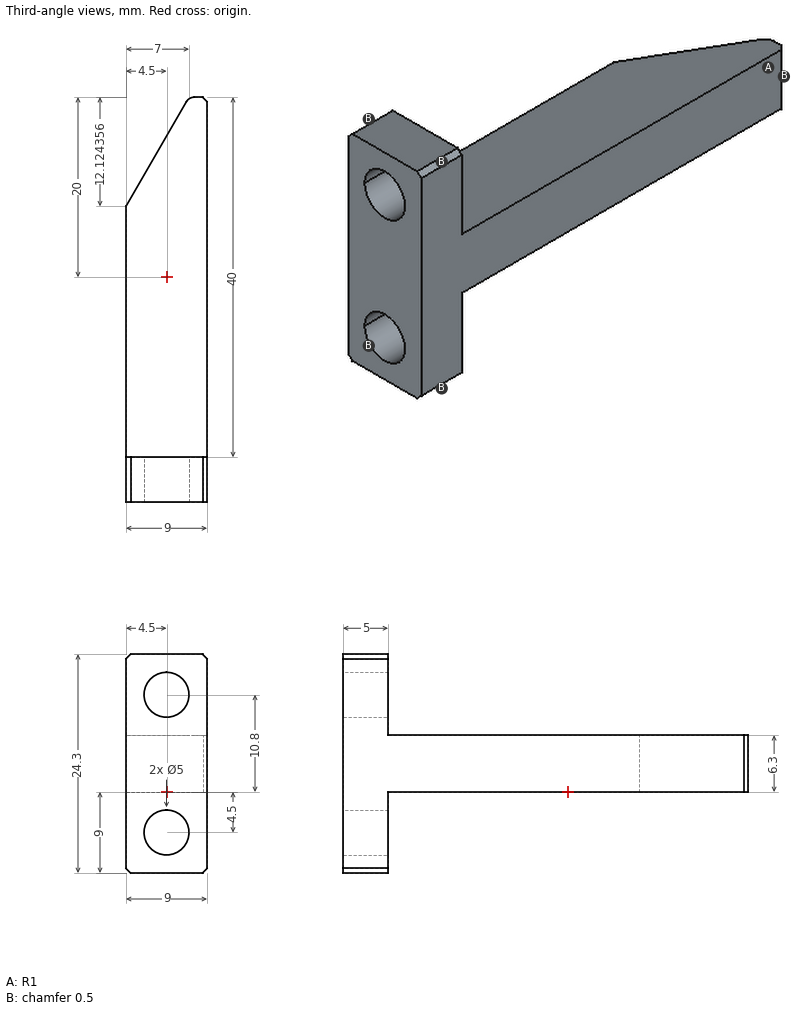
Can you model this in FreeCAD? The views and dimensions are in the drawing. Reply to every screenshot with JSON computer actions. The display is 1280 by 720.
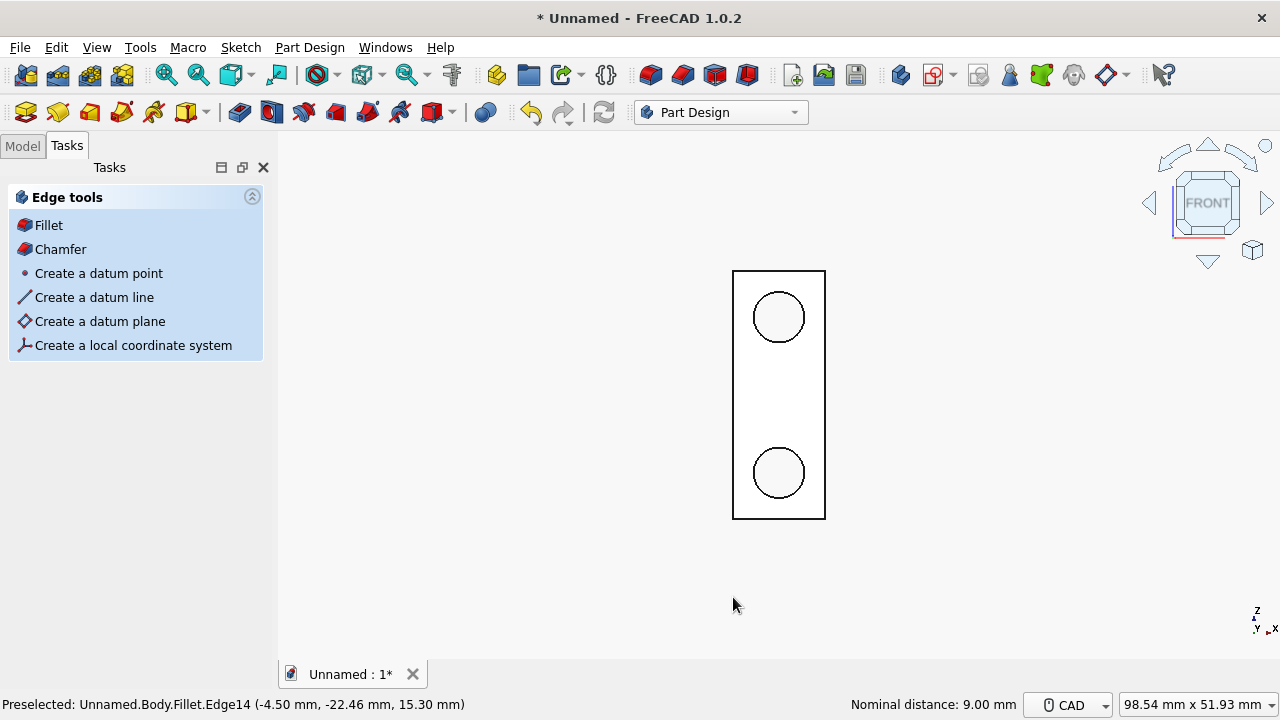
{"action": "key", "text": "3"}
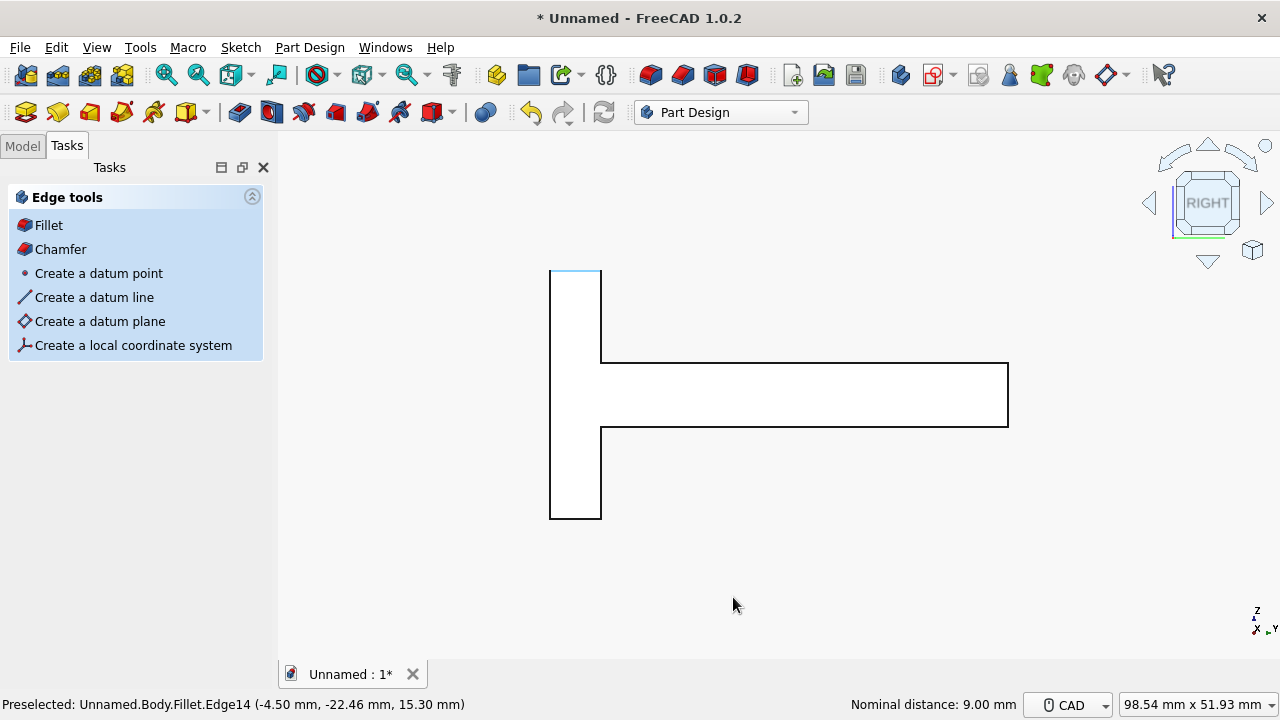
{"action": "left_click", "coordinate": [576, 518], "text": "ctrl"}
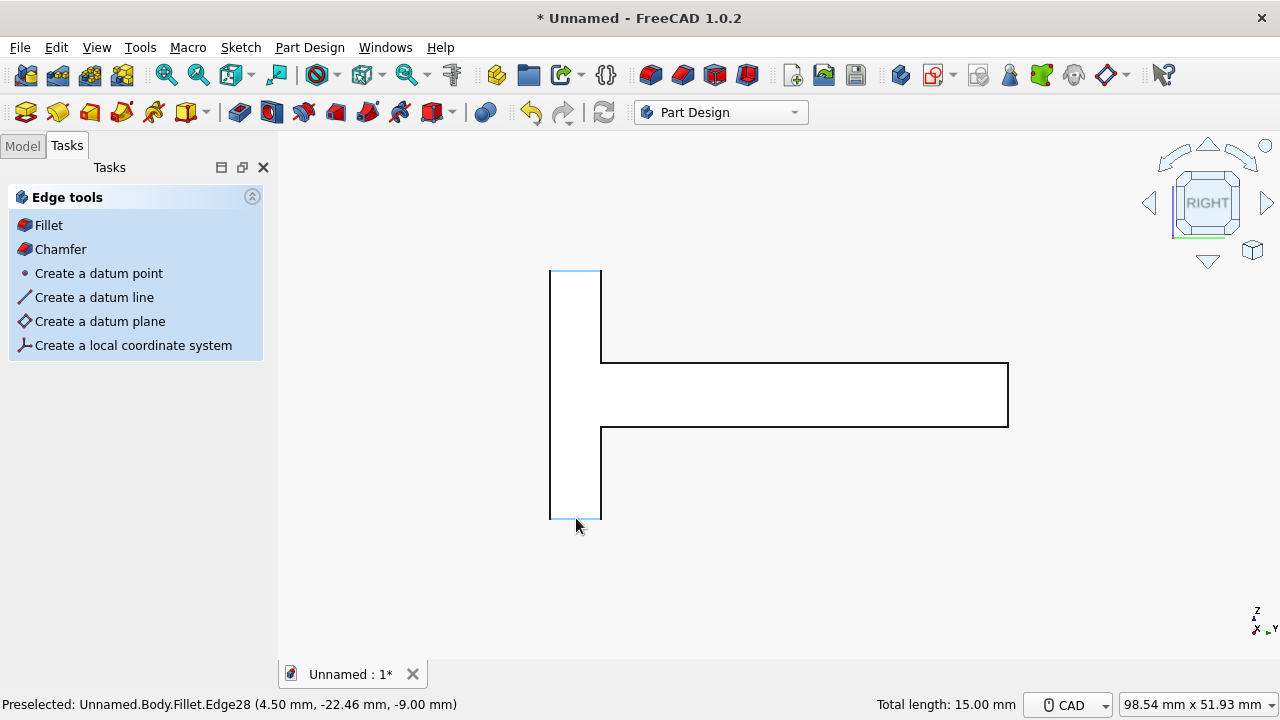
{"action": "left_click", "coordinate": [1008, 394], "text": "ctrl"}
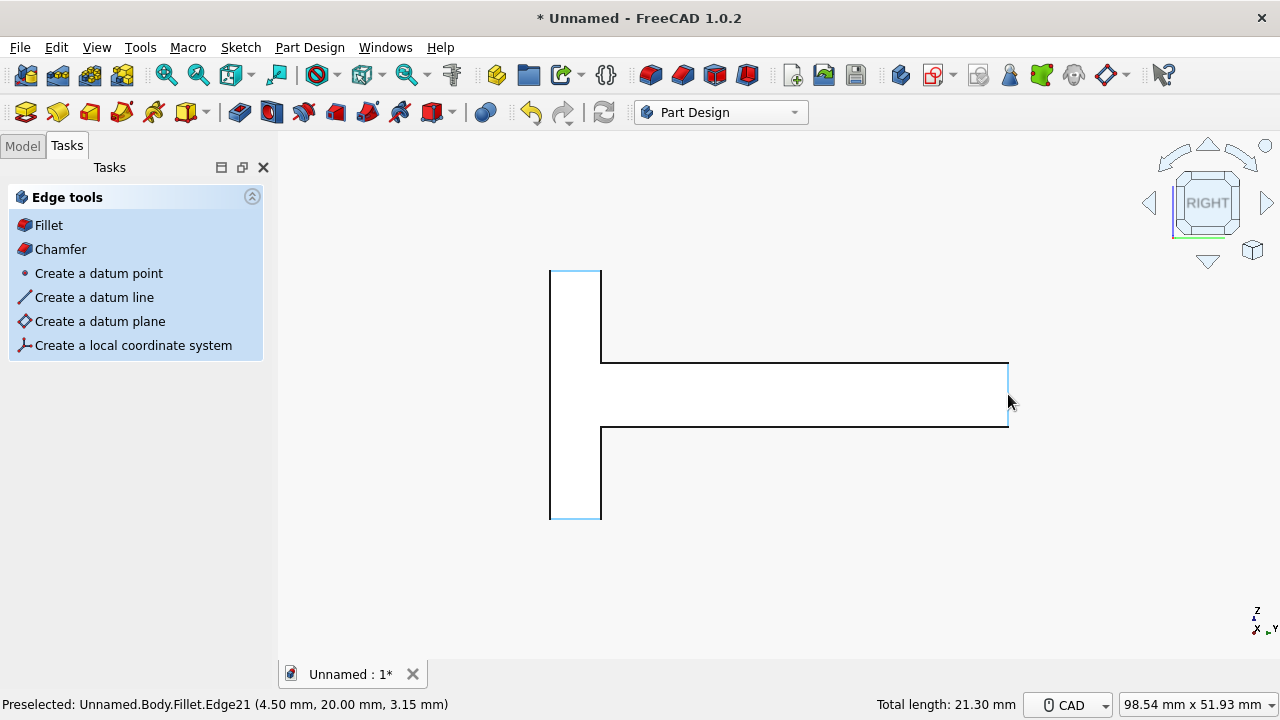
{"action": "key", "text": "5"}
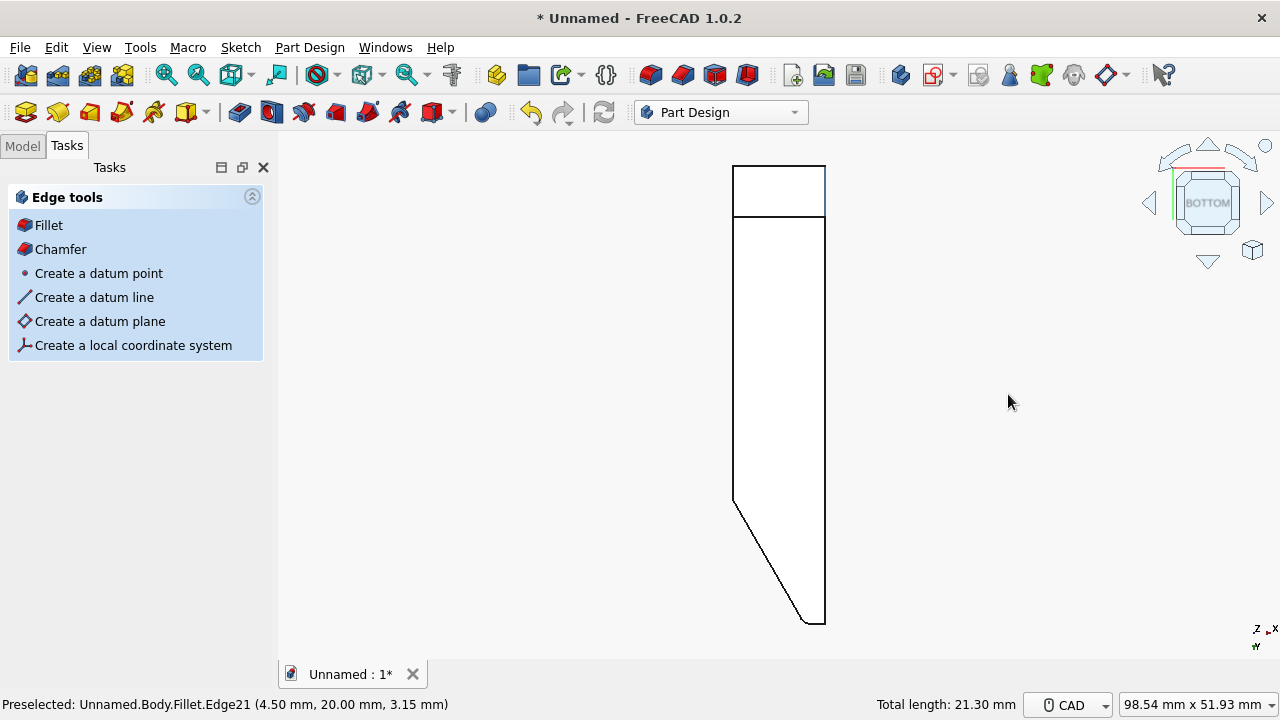
{"action": "left_click", "coordinate": [733, 191], "text": "ctrl"}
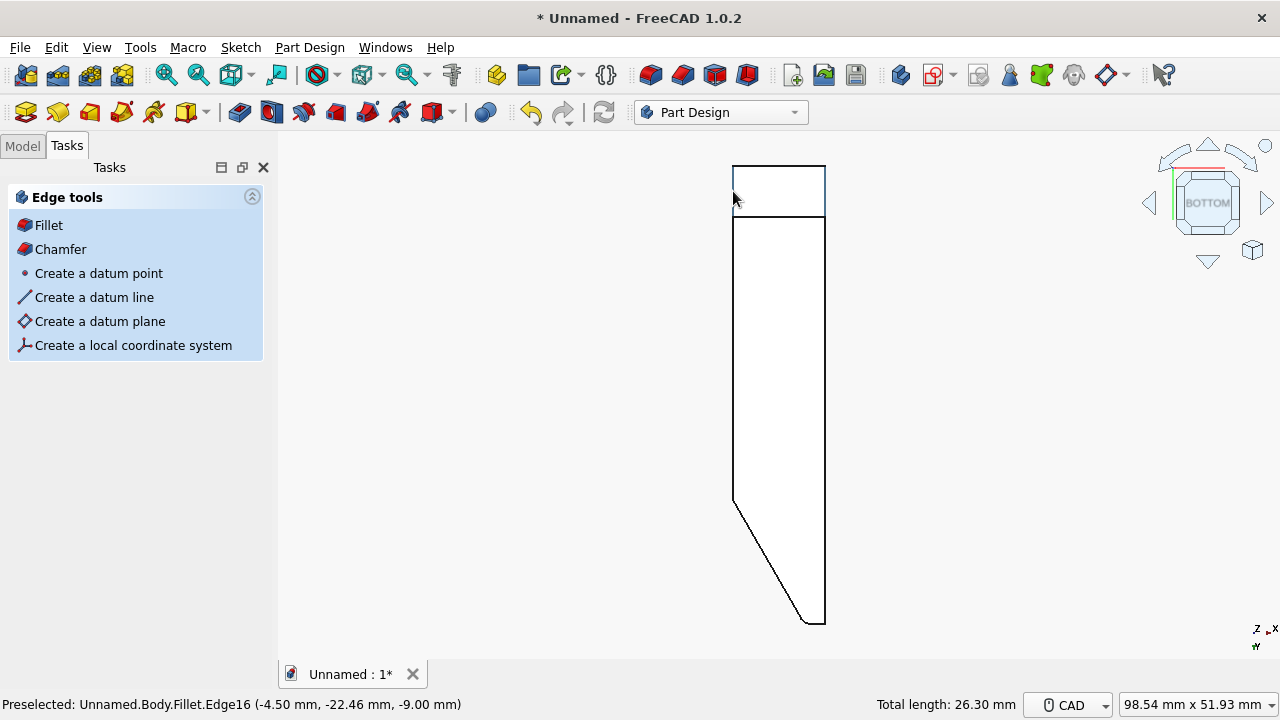
{"action": "left_click", "coordinate": [684, 76]}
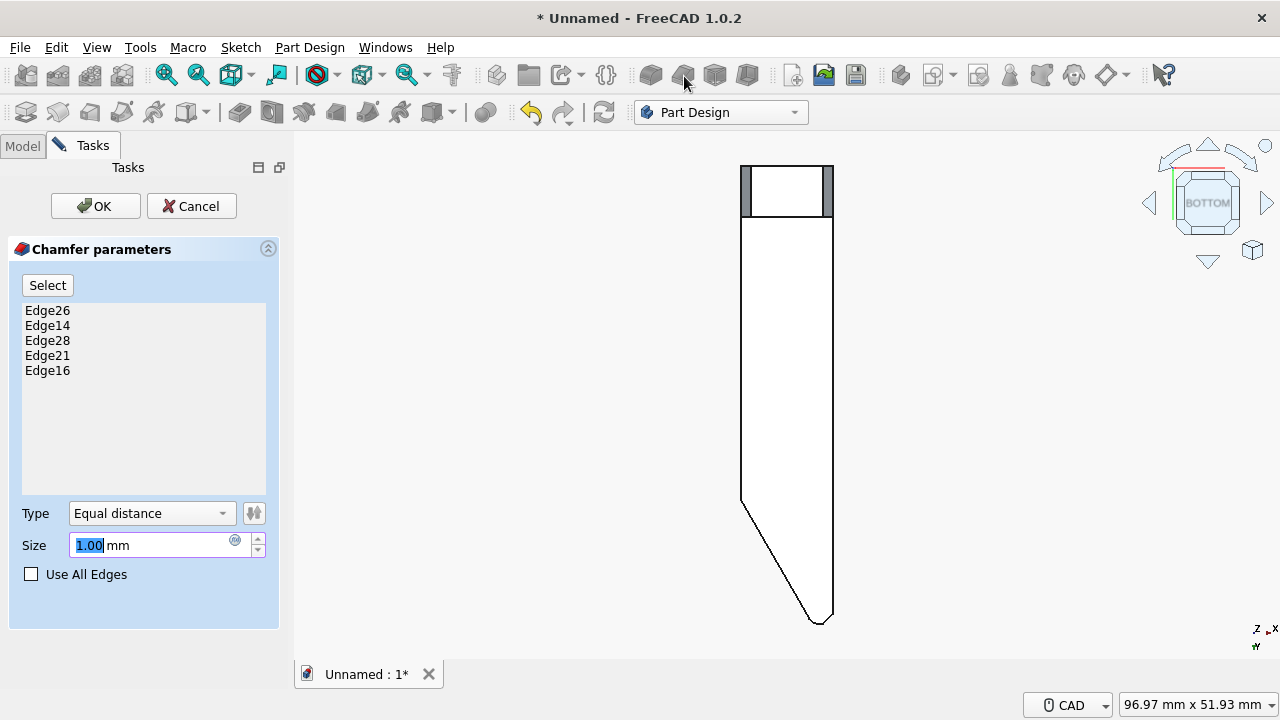
{"action": "type", "text": "0.5"}
{"action": "key", "text": "Tab"}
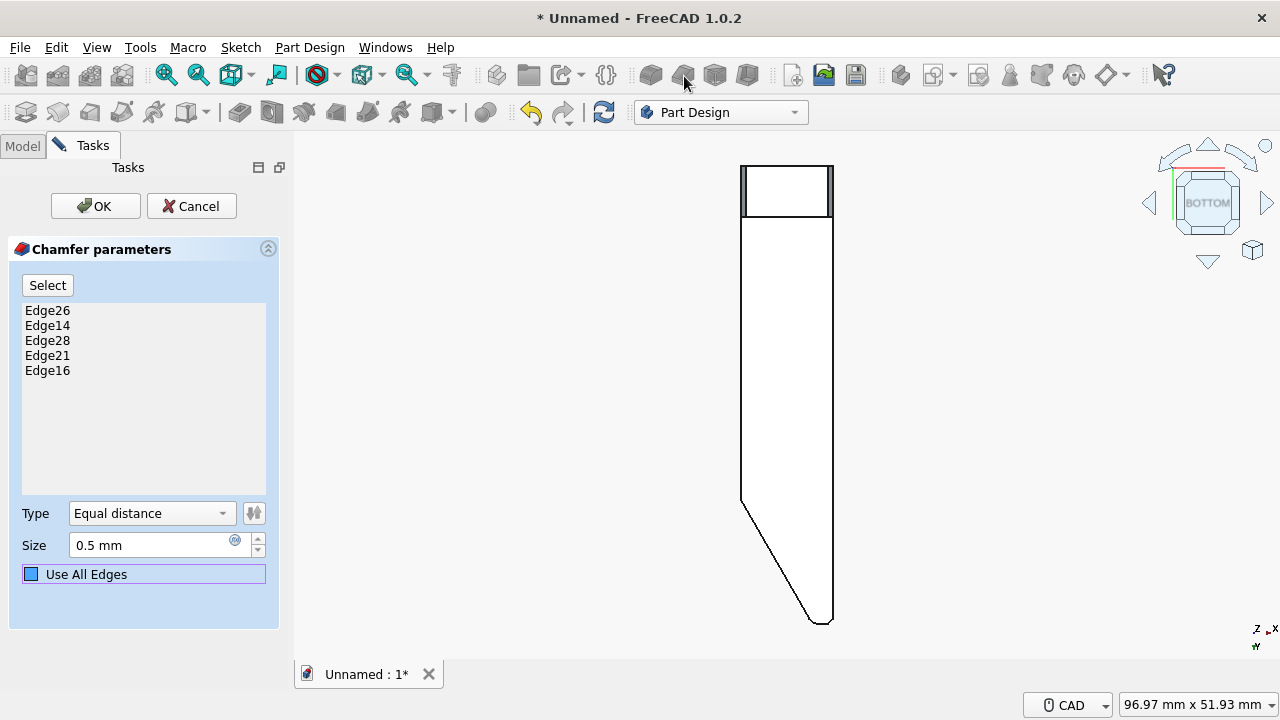
{"action": "left_click", "coordinate": [96, 206]}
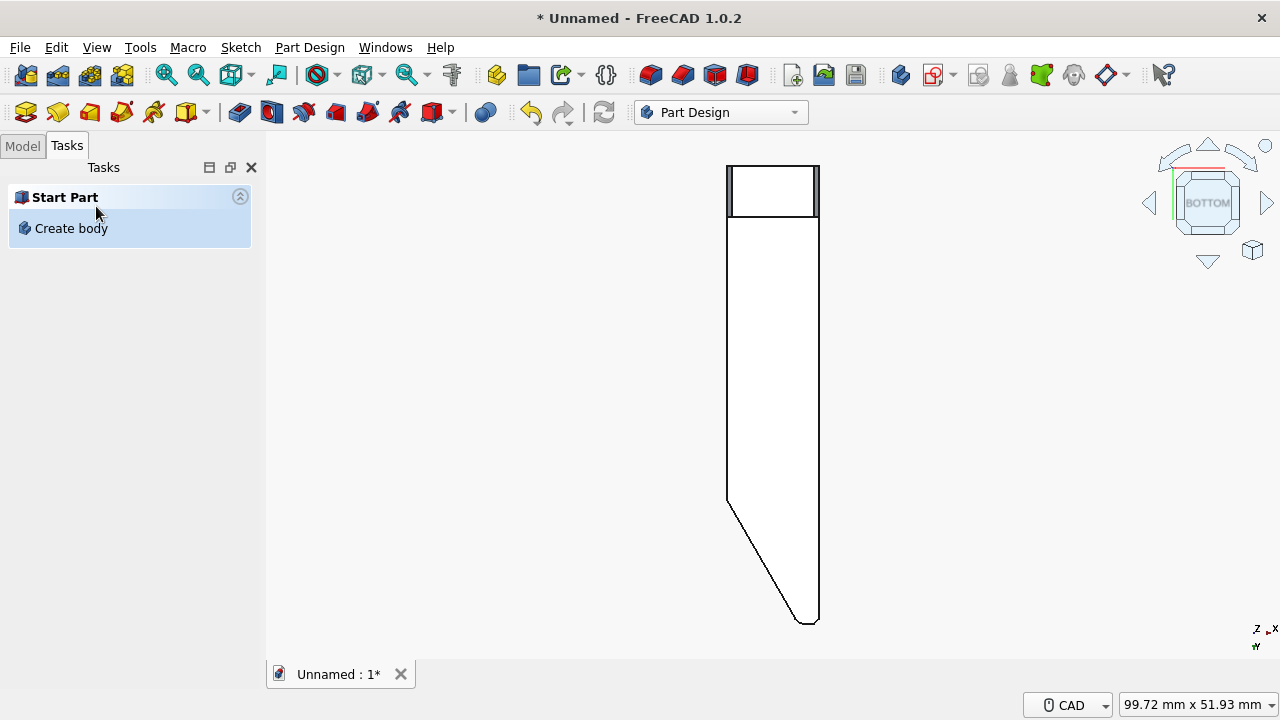
{"action": "key", "text": "0"}